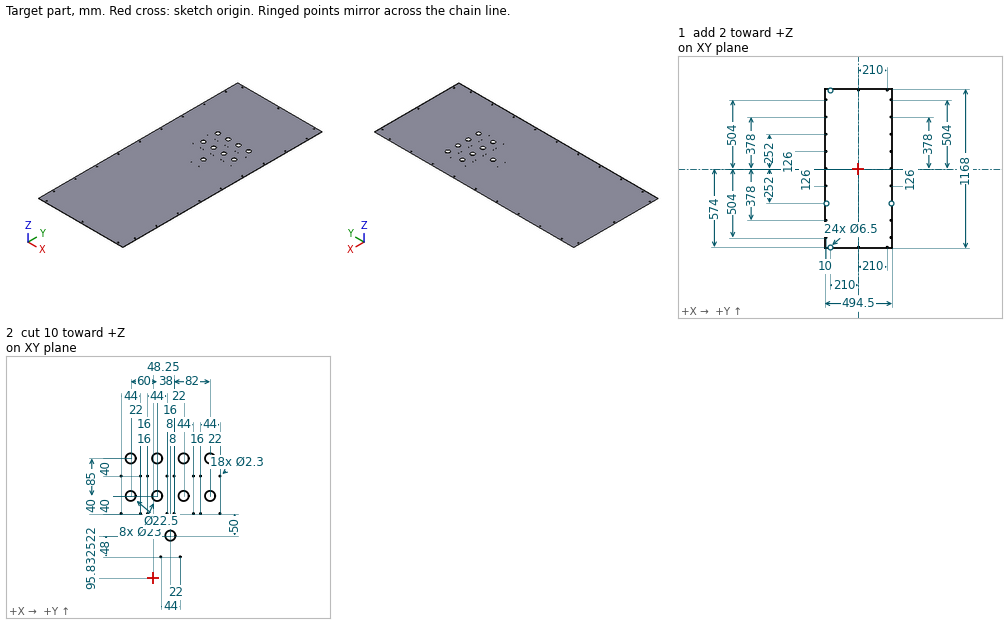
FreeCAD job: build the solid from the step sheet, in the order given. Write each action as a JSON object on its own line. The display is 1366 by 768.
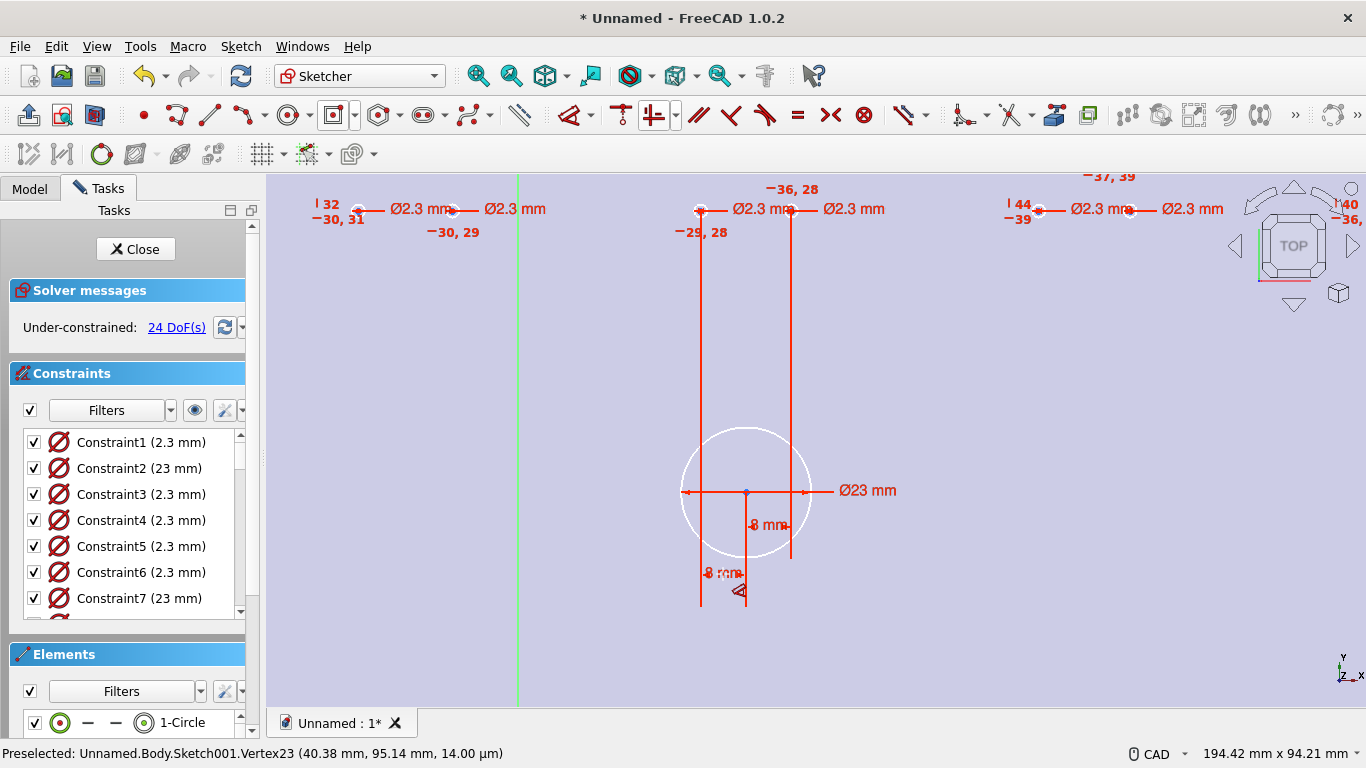
{"action": "scroll", "coordinate": [748, 493], "scroll_direction": "down", "scroll_amount": 8}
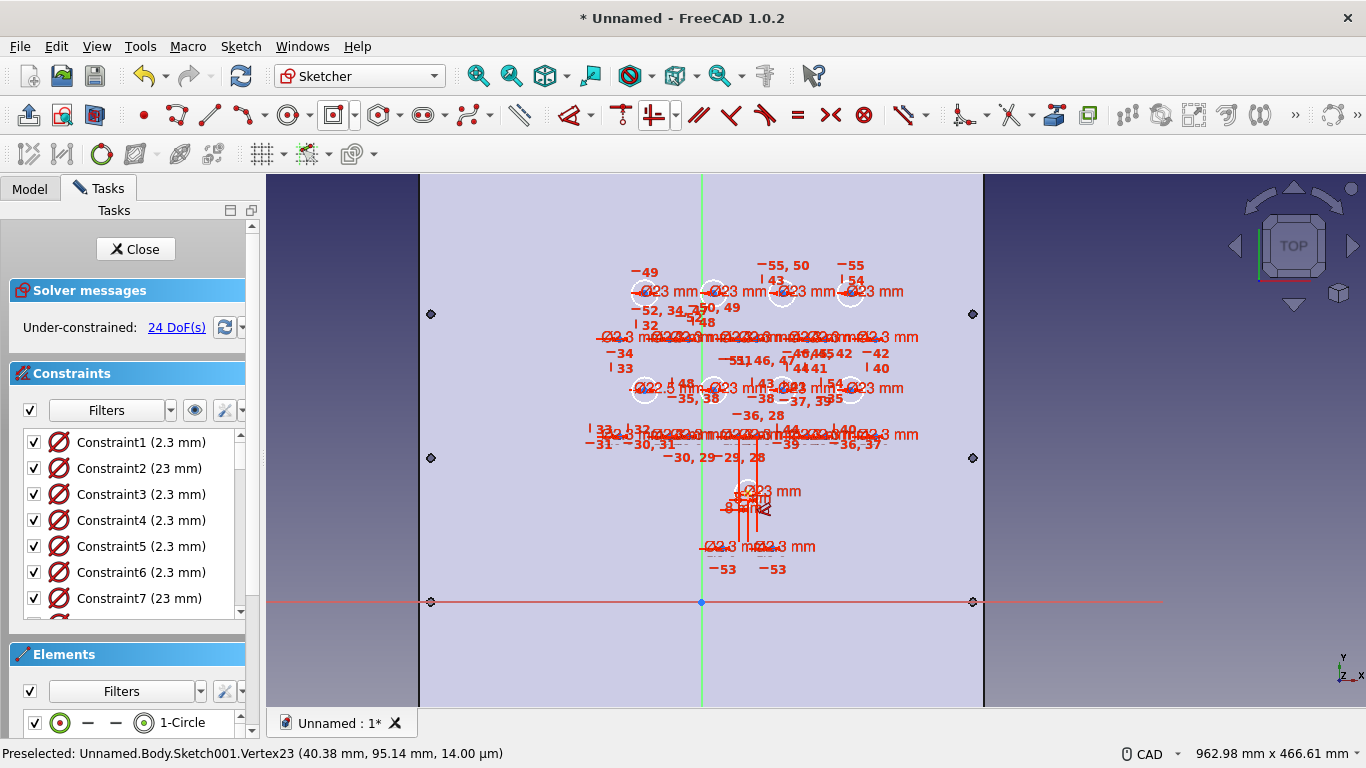
{"action": "left_click", "coordinate": [757, 437]}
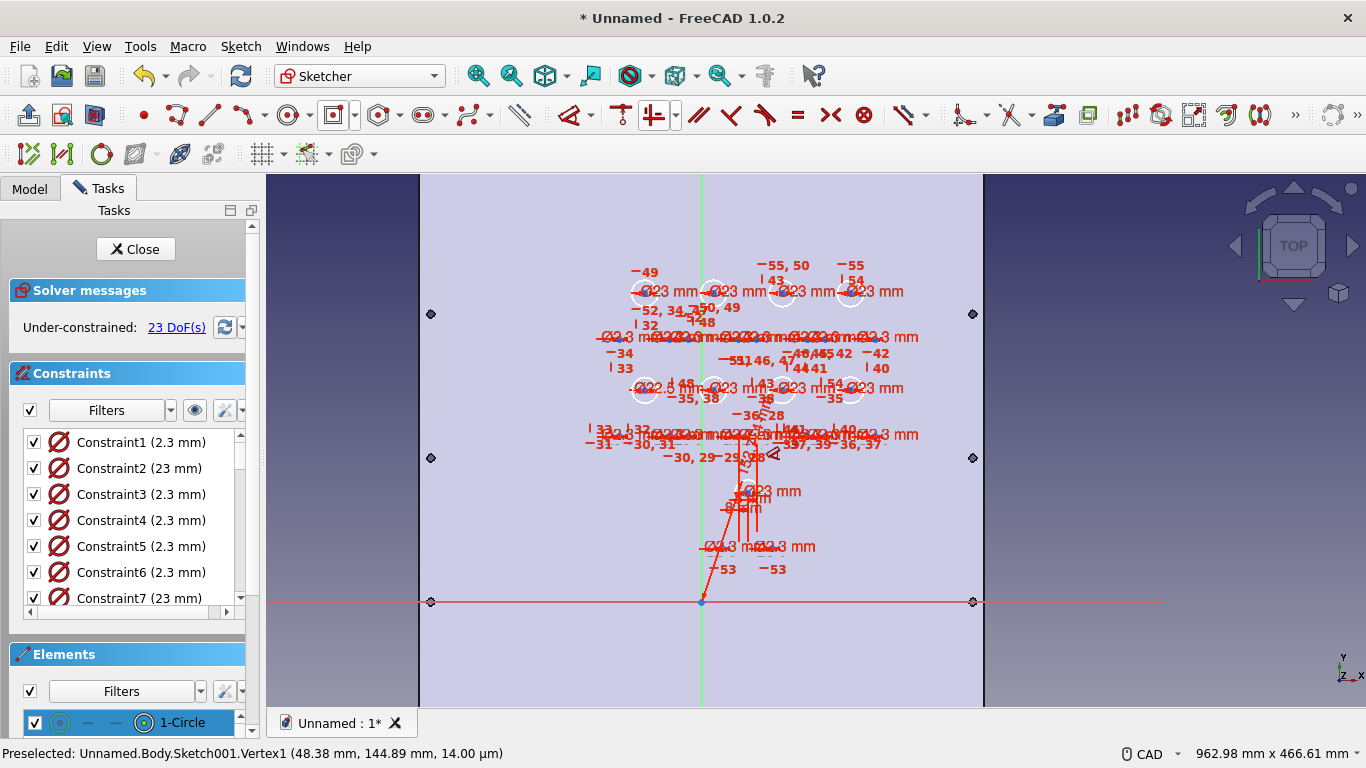
{"action": "left_click", "coordinate": [714, 390]}
{"action": "left_click", "coordinate": [735, 356]}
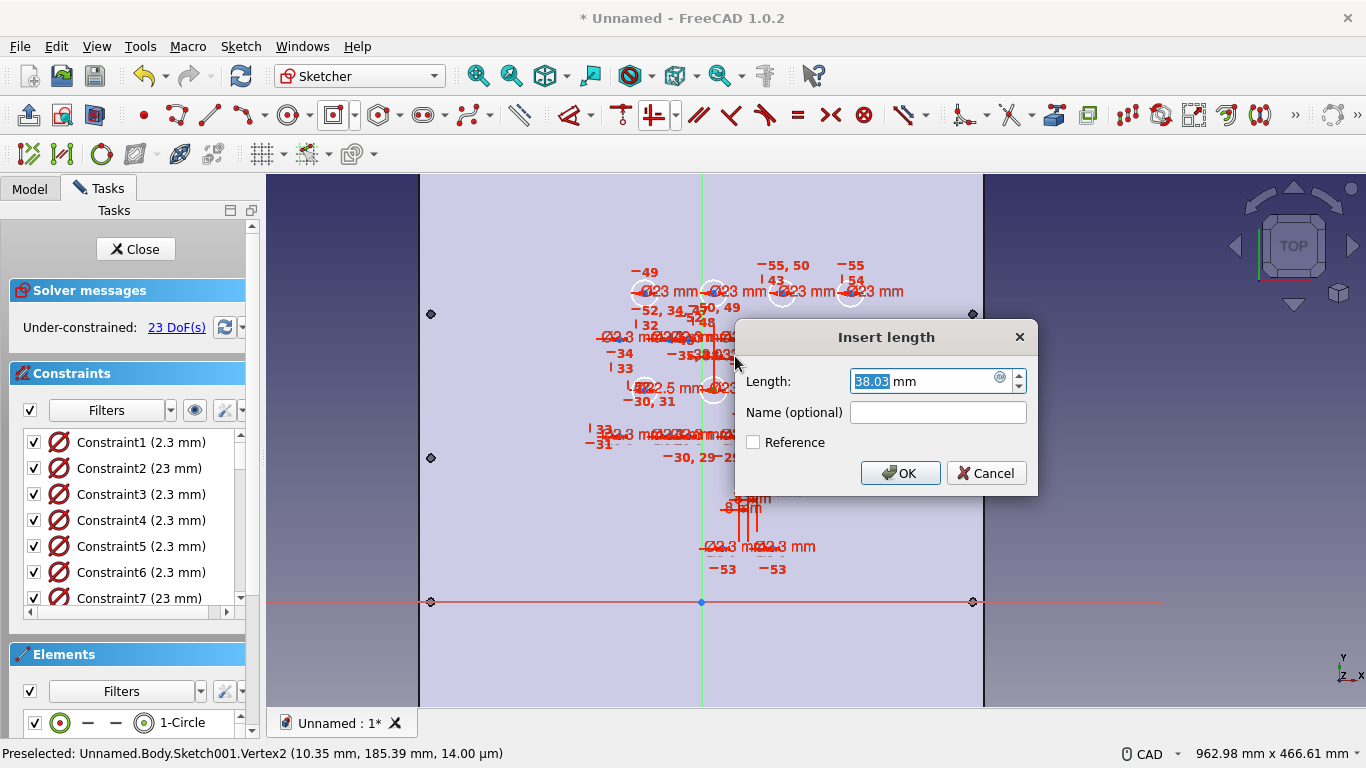
{"action": "type", "text": "38"}
{"action": "key", "text": "Return"}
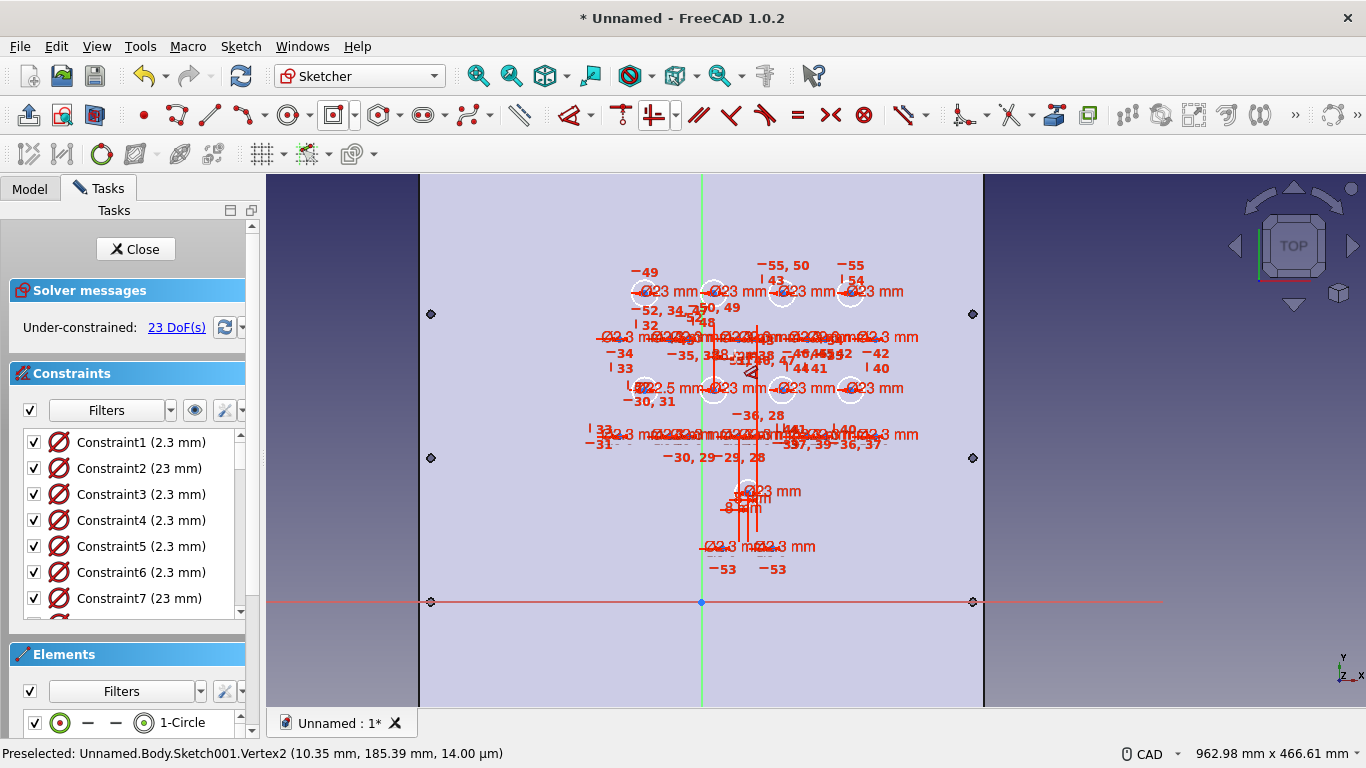
{"action": "left_click", "coordinate": [757, 437]}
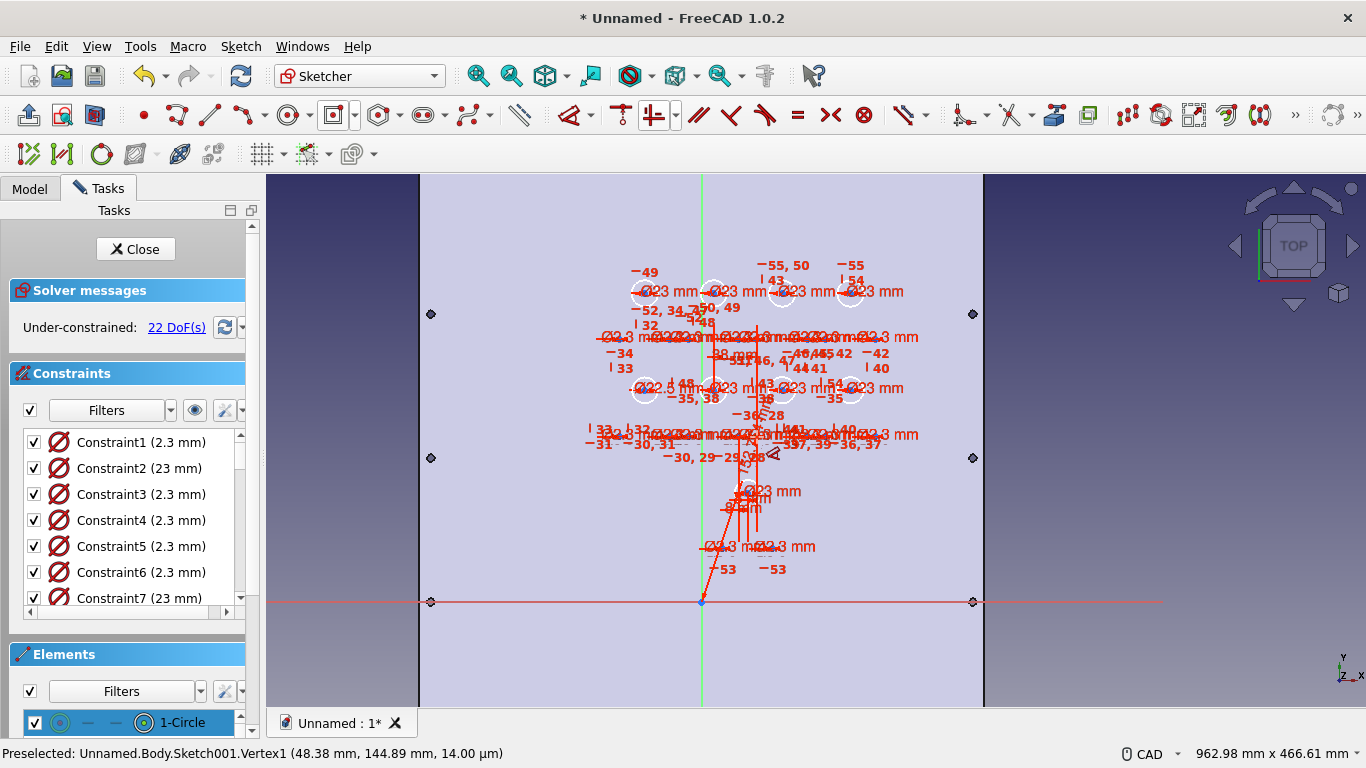
{"action": "left_click", "coordinate": [714, 390]}
{"action": "left_click", "coordinate": [680, 413]}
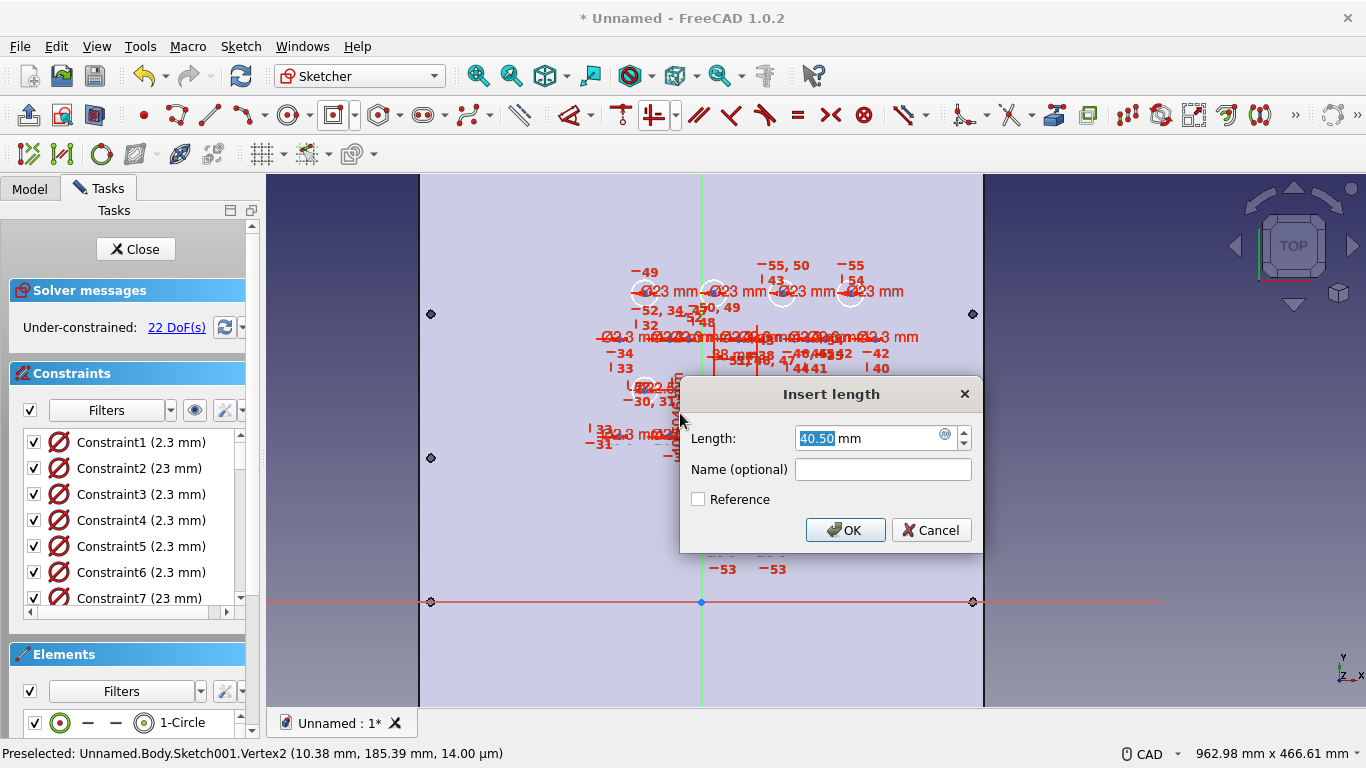
{"action": "type", "text": "40"}
{"action": "key", "text": "Return"}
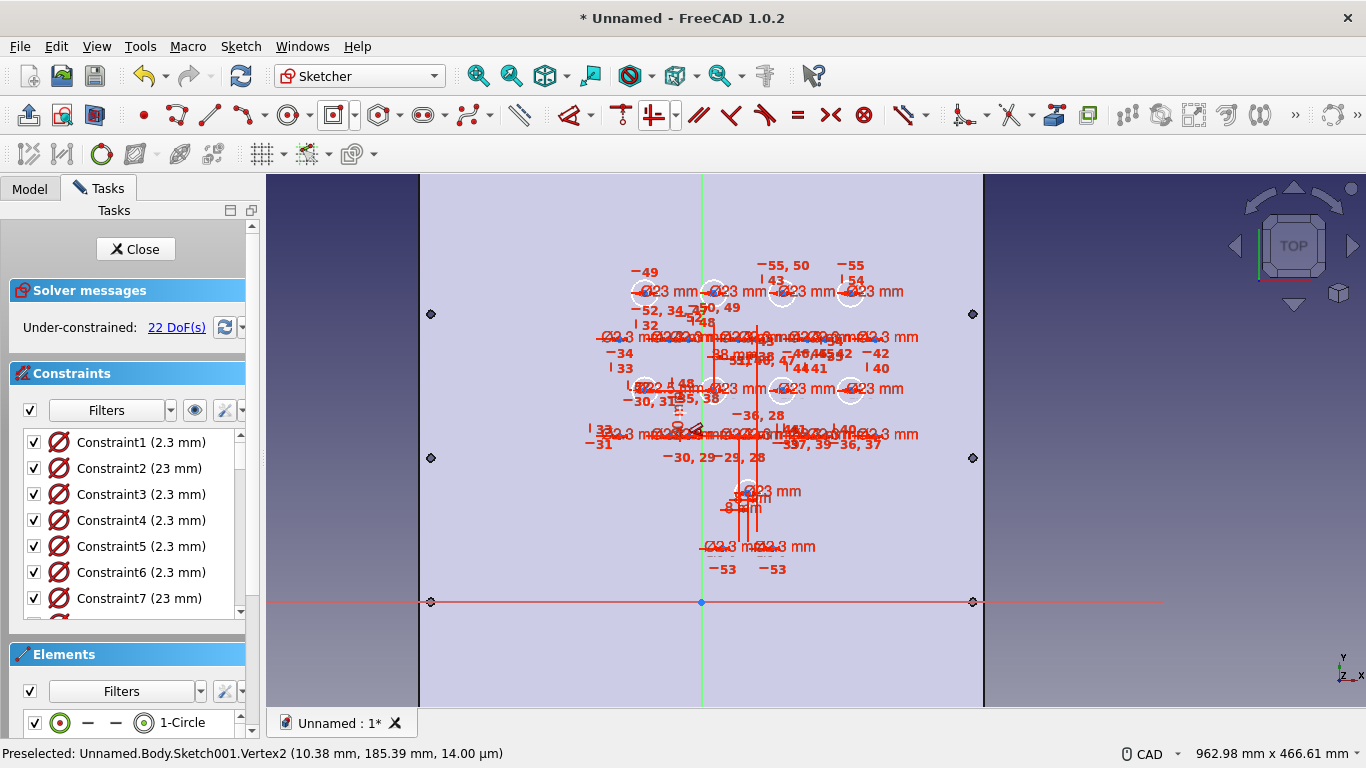
{"action": "left_click", "coordinate": [739, 436]}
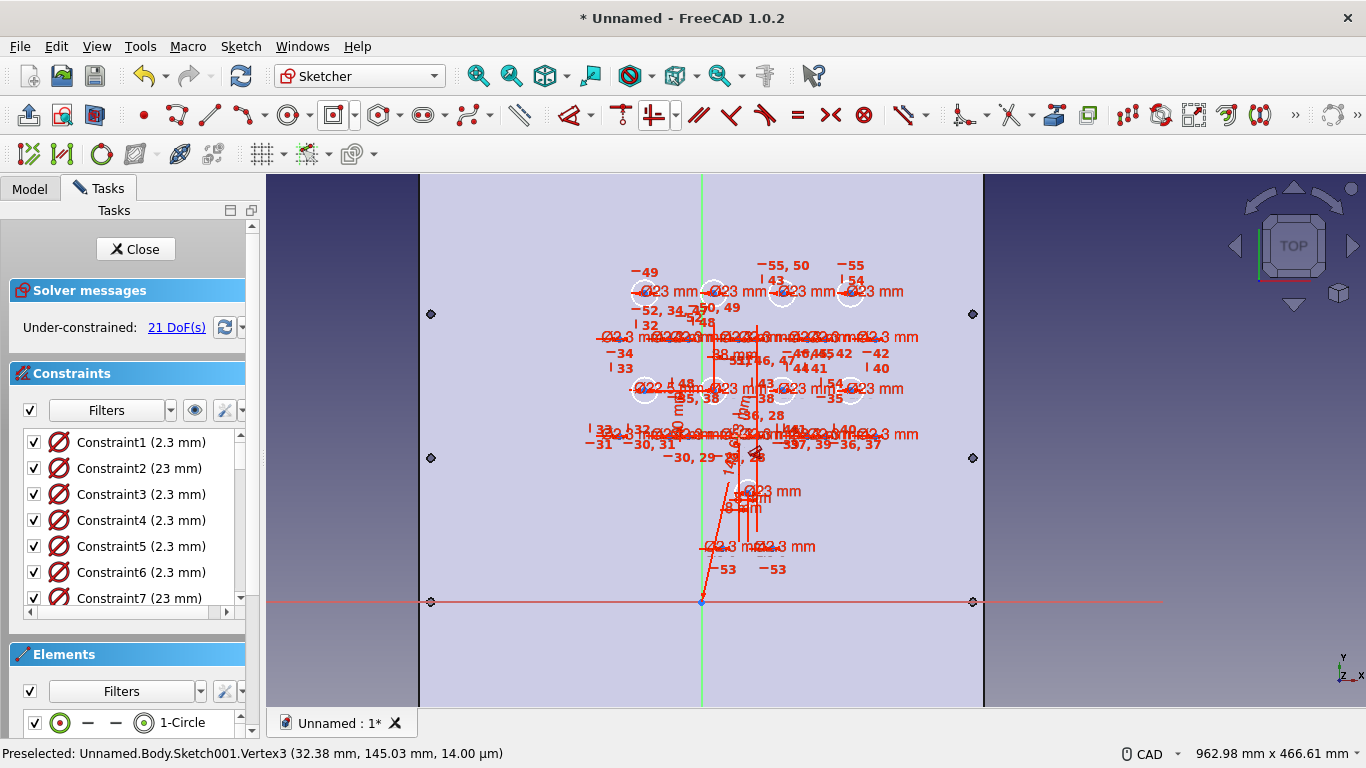
{"action": "left_click", "coordinate": [689, 436]}
{"action": "left_click", "coordinate": [725, 470]}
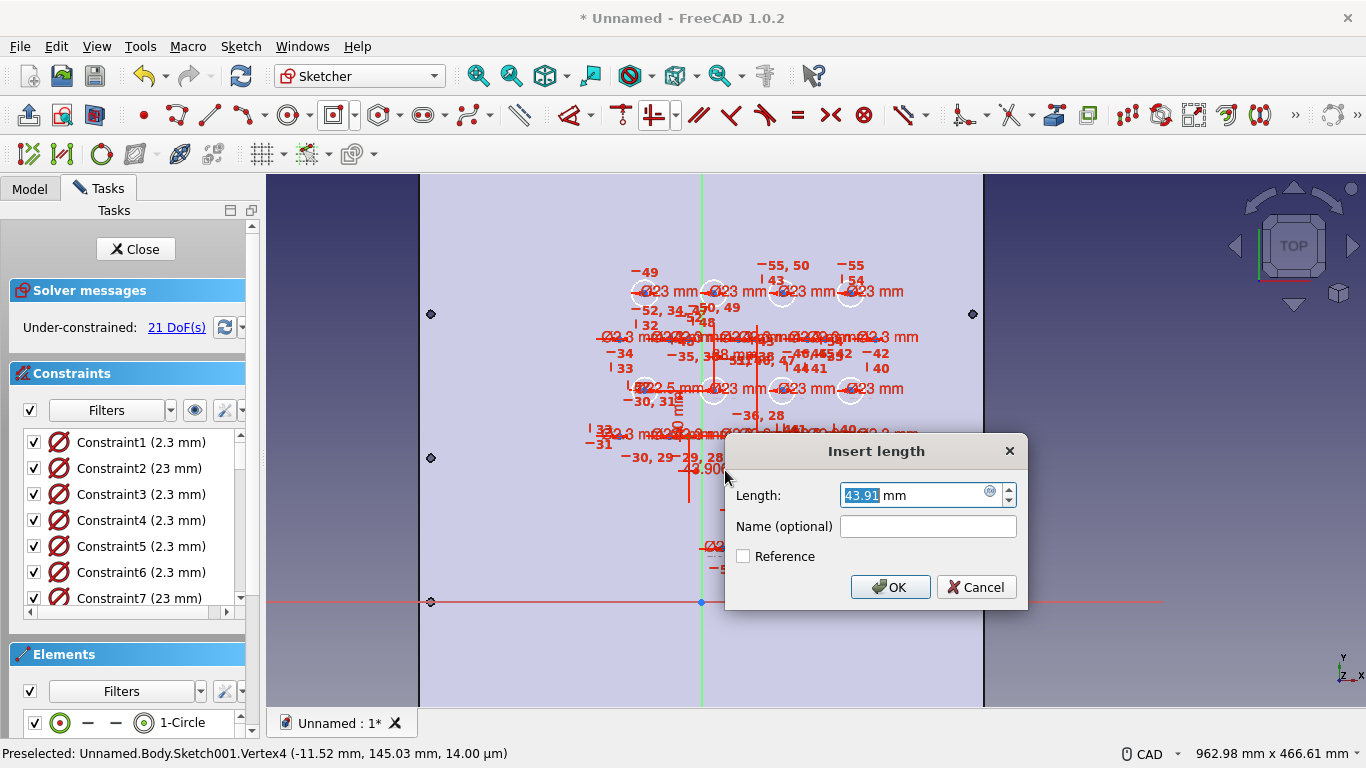
{"action": "type", "text": "44"}
{"action": "key", "text": "Return"}